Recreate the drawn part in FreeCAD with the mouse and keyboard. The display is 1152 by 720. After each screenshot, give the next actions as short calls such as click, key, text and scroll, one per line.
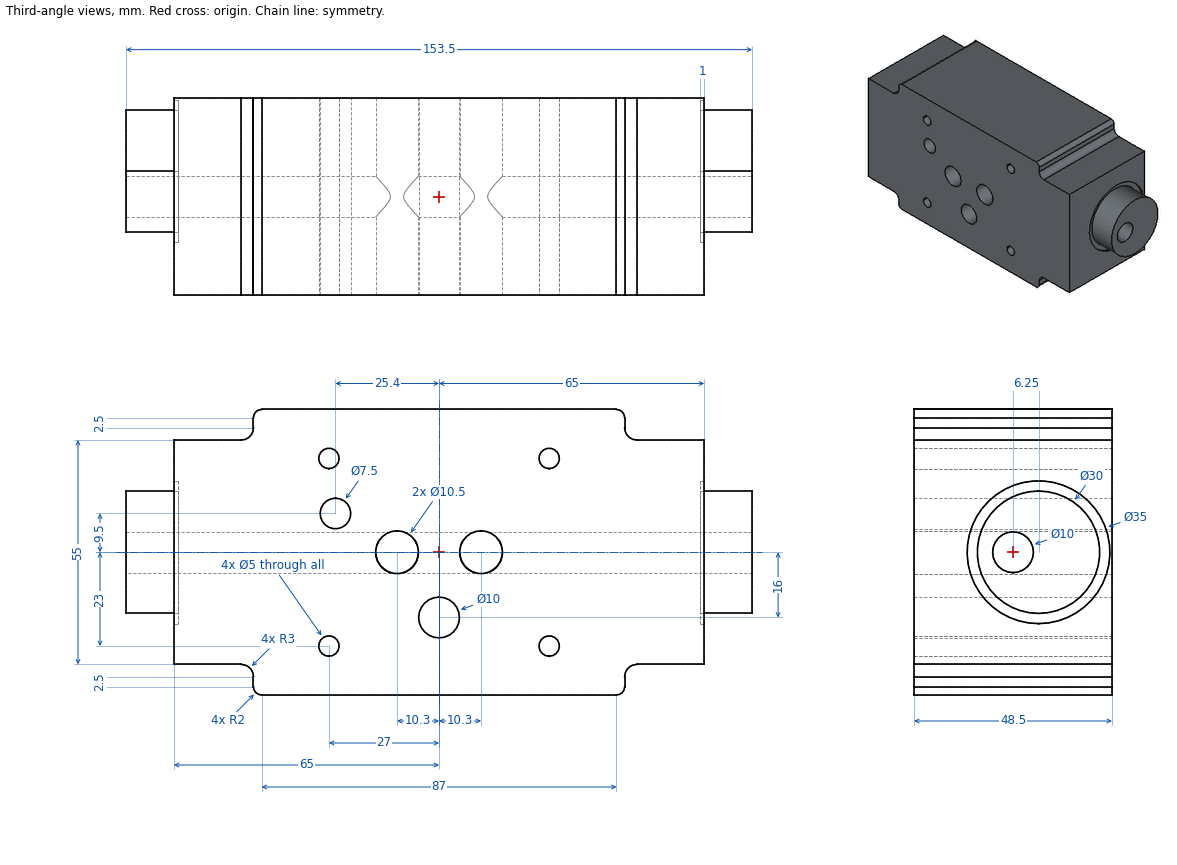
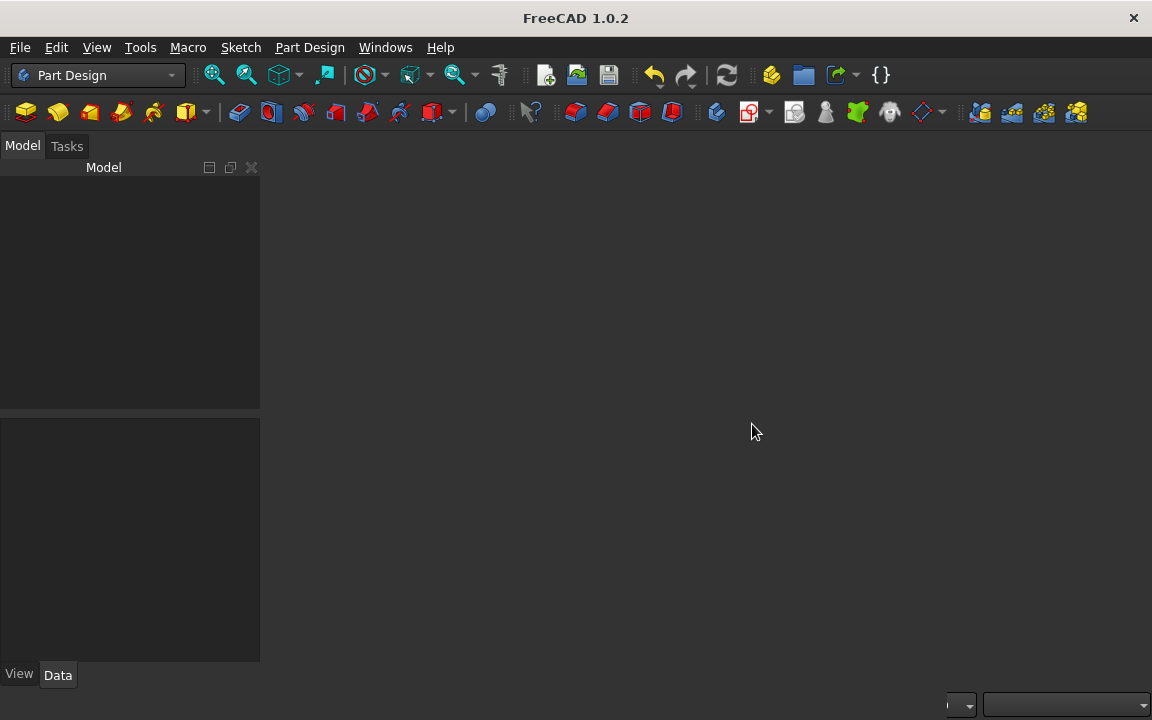
click(546, 76)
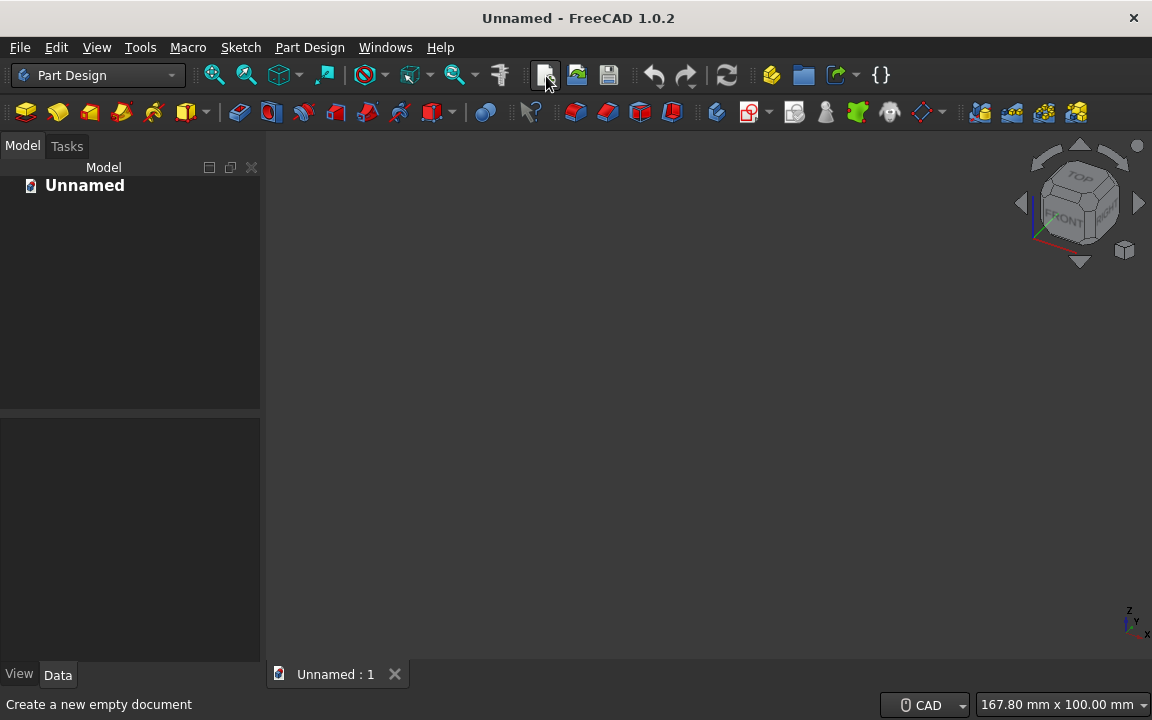
click(750, 112)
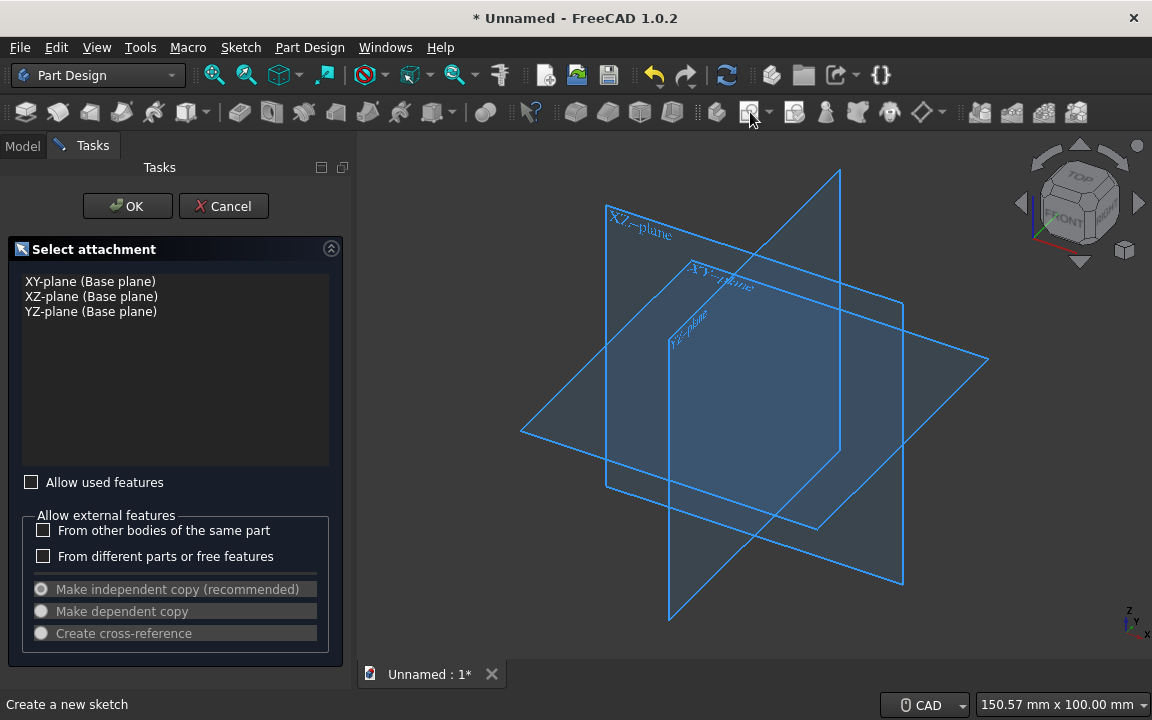
click(82, 296)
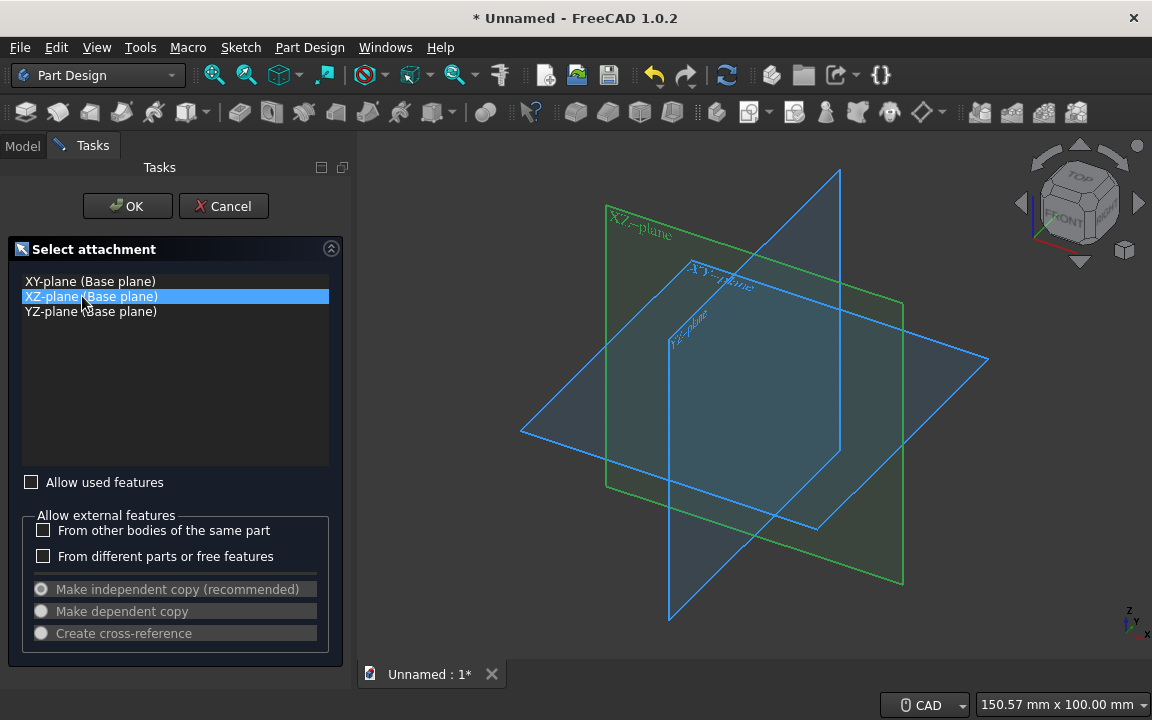
click(128, 206)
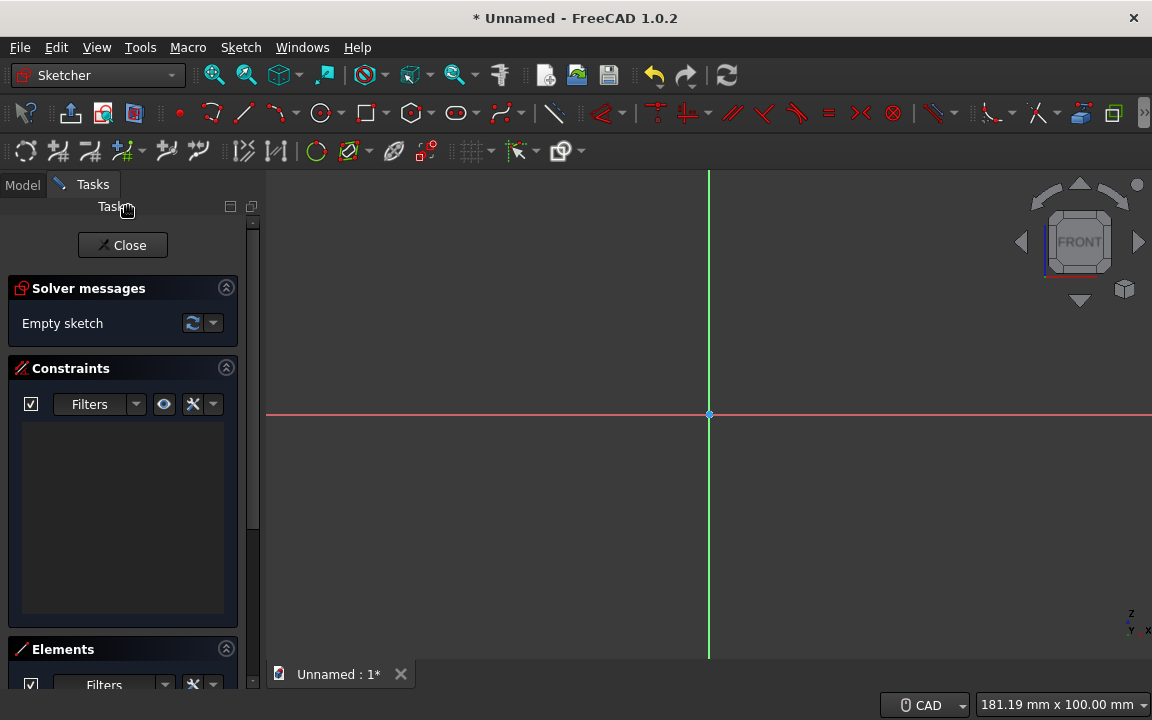
scroll(331, 415, down, 1)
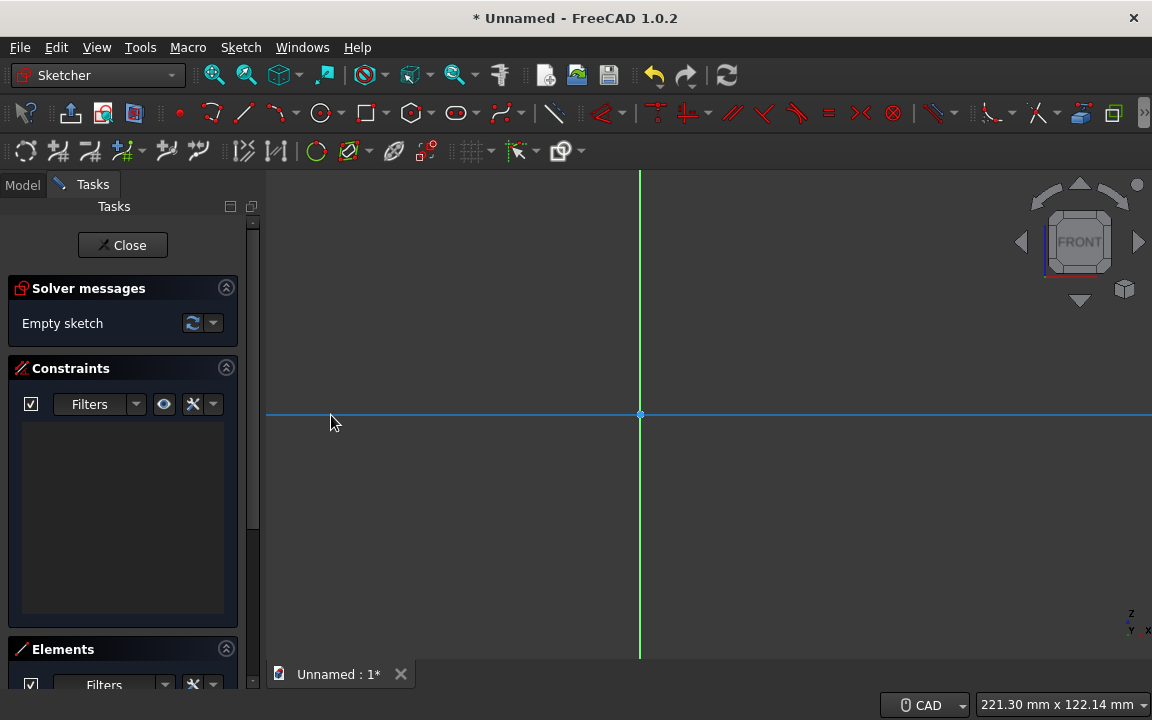
click(244, 114)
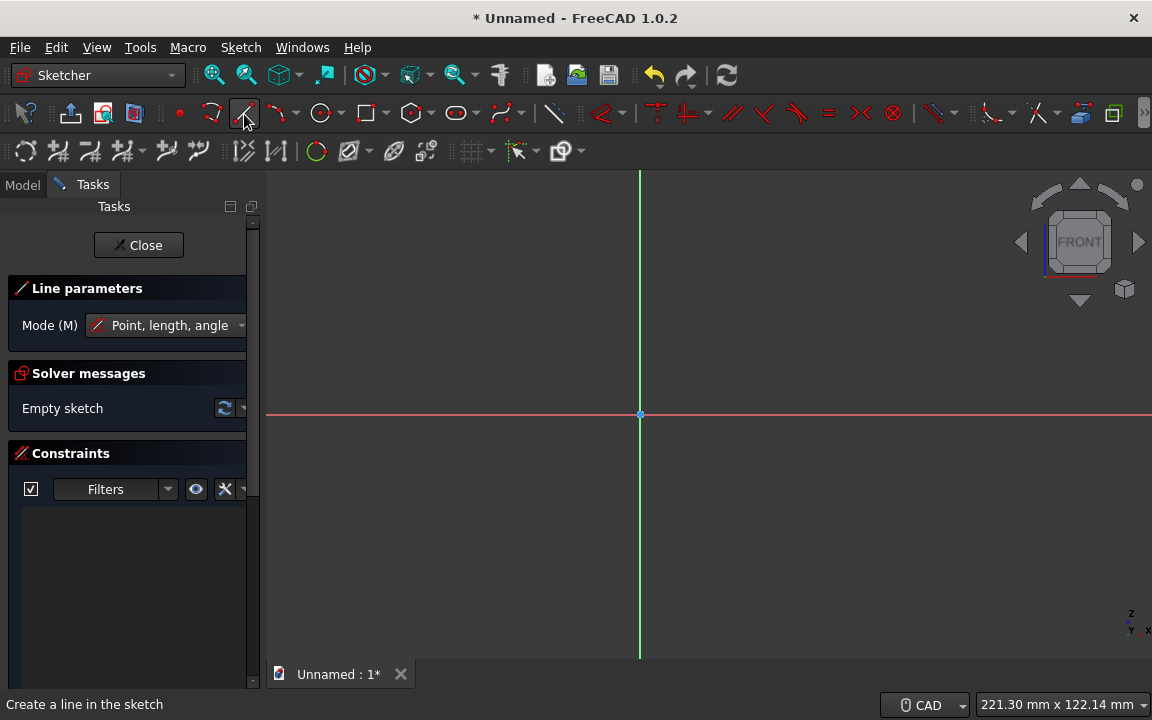
click(815, 555)
click(466, 555)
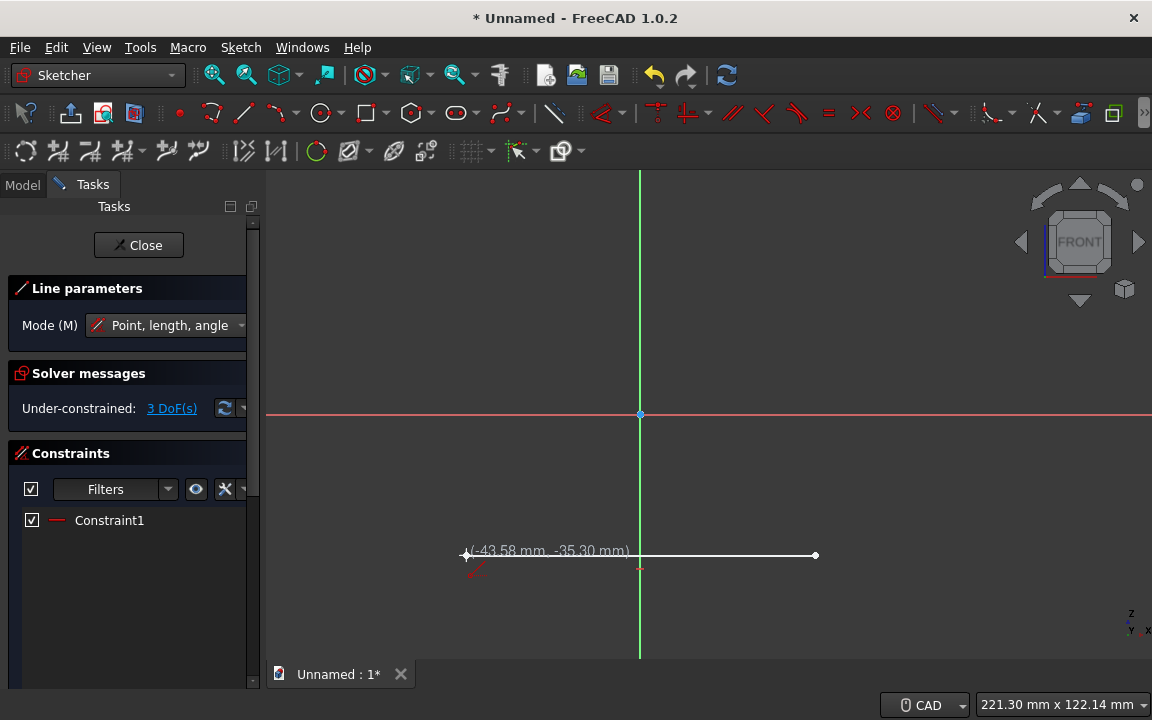
scroll(458, 547, up, 2)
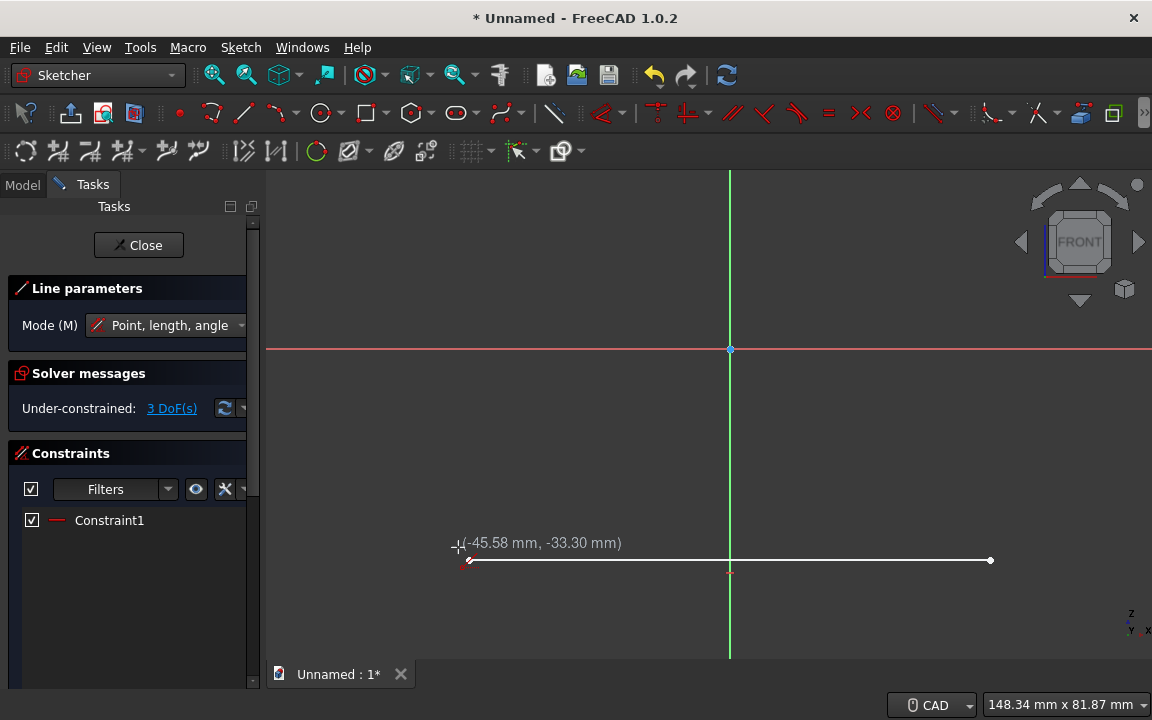
click(458, 546)
click(458, 531)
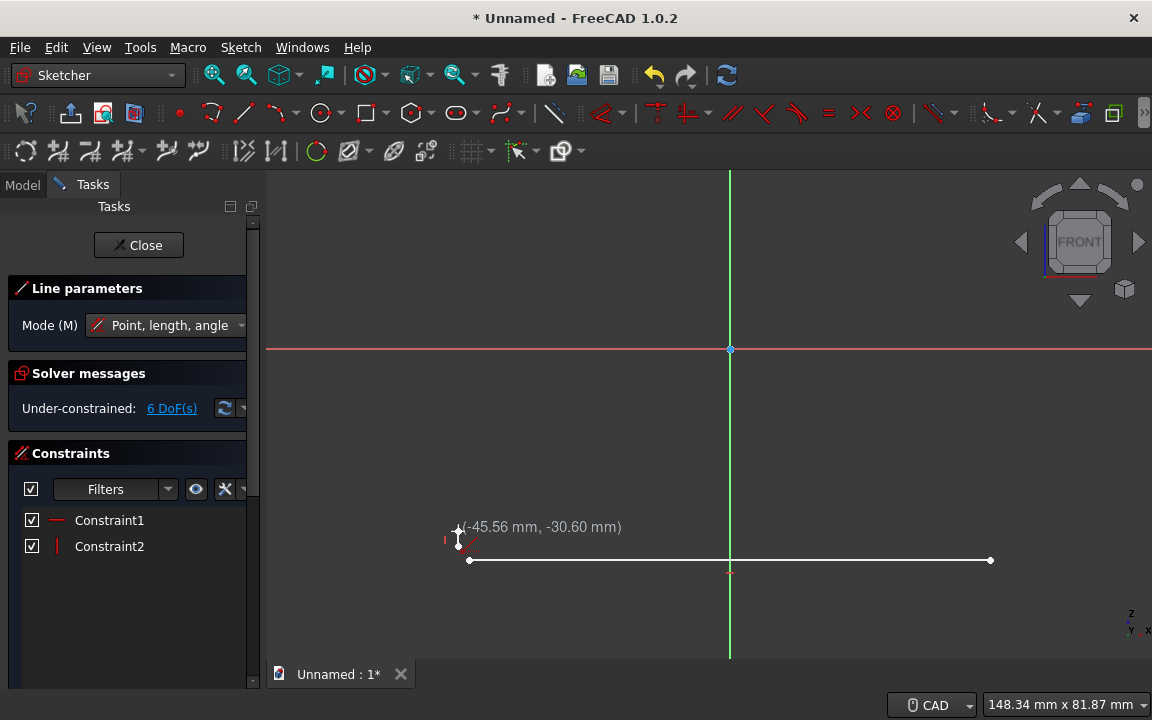
click(212, 114)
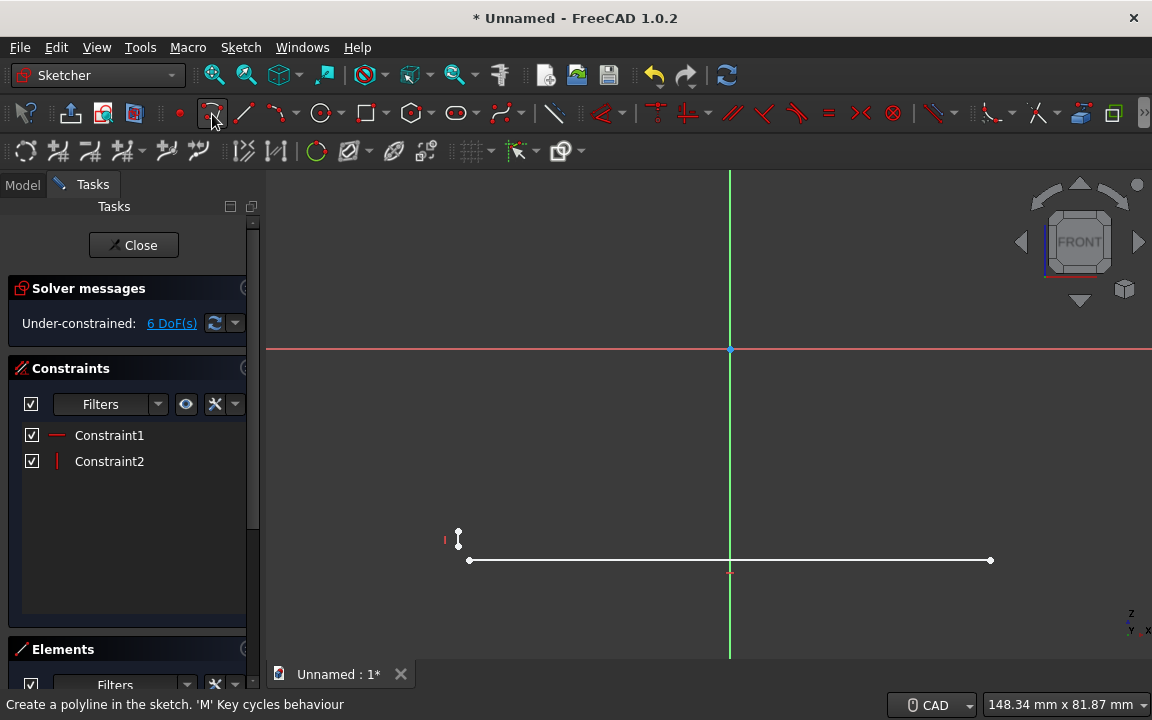
click(440, 513)
click(342, 513)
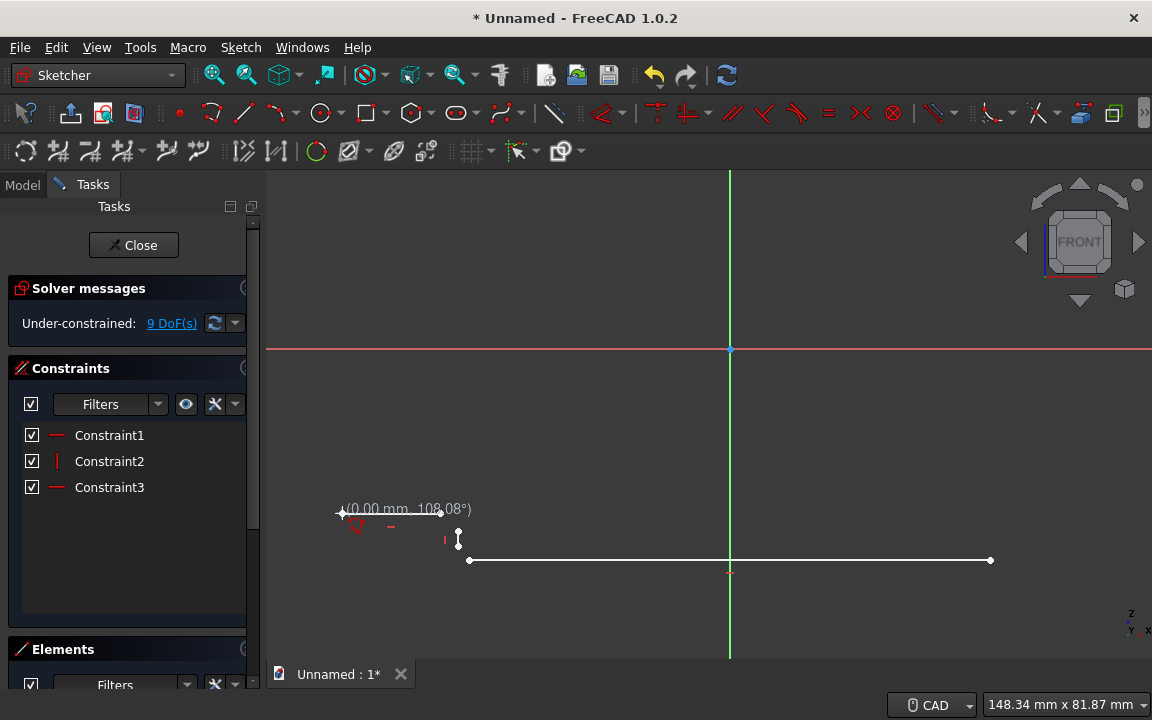
scroll(458, 547, down, 2)